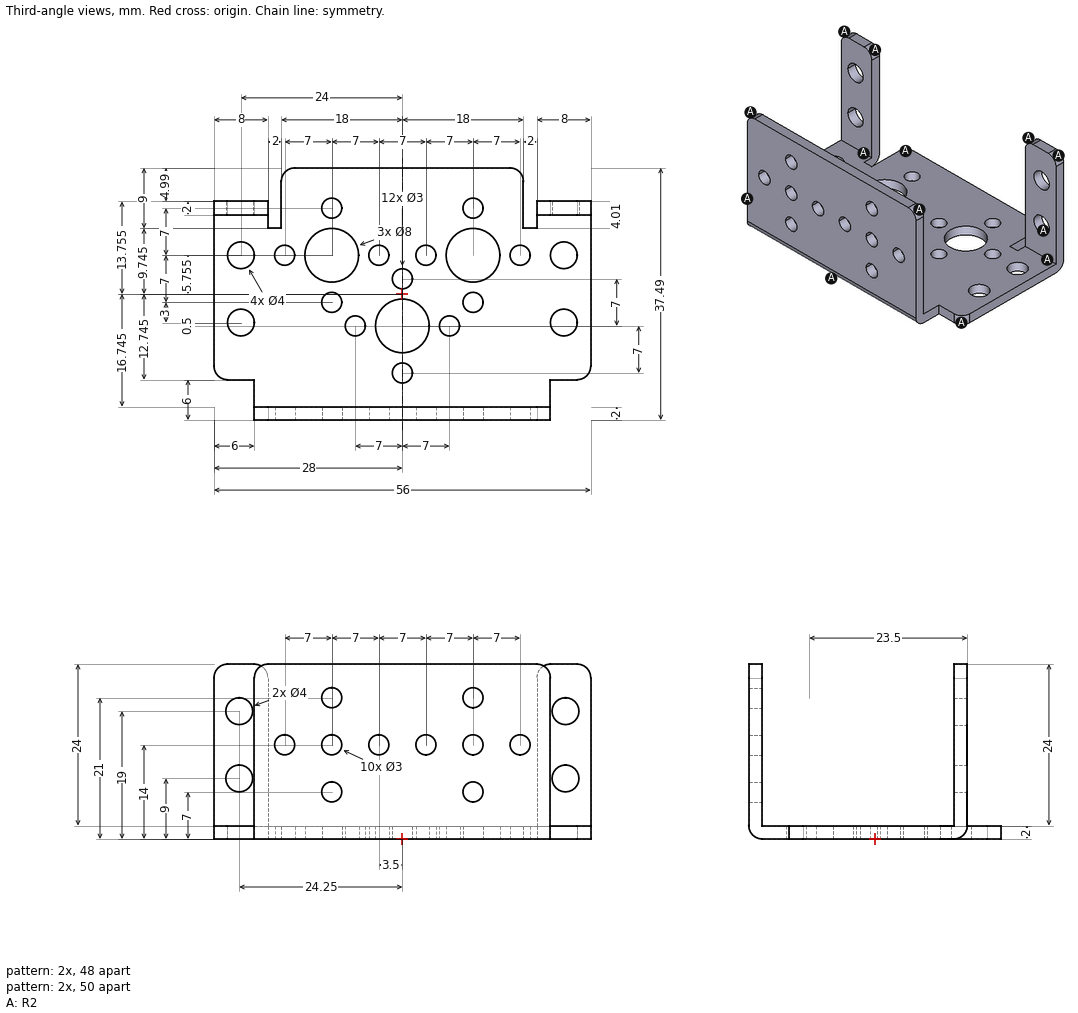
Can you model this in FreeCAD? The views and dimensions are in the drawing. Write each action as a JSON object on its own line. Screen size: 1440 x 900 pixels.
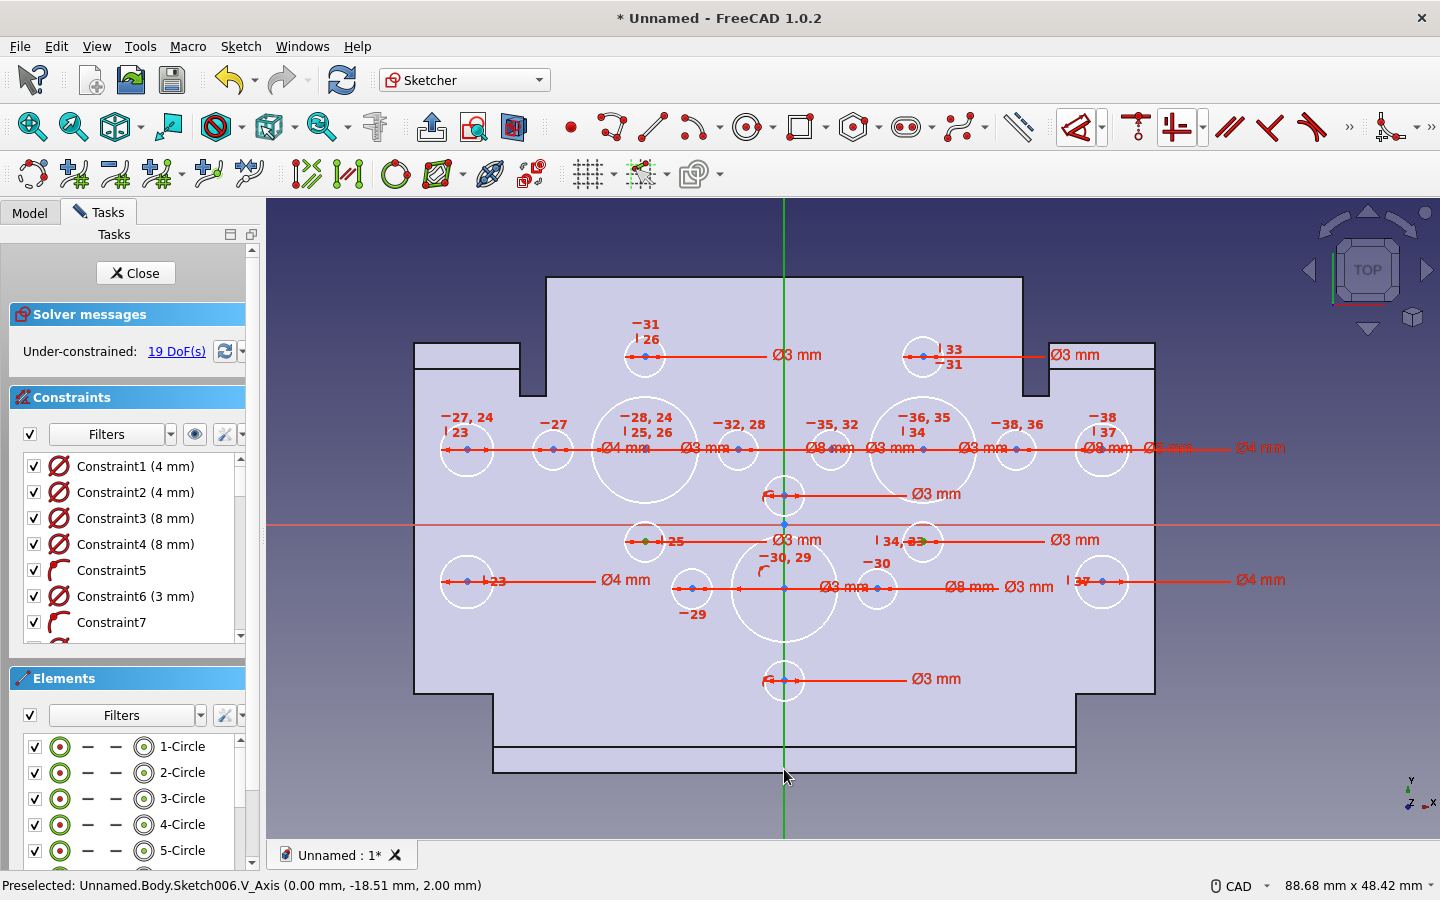
{"action": "key", "text": "s"}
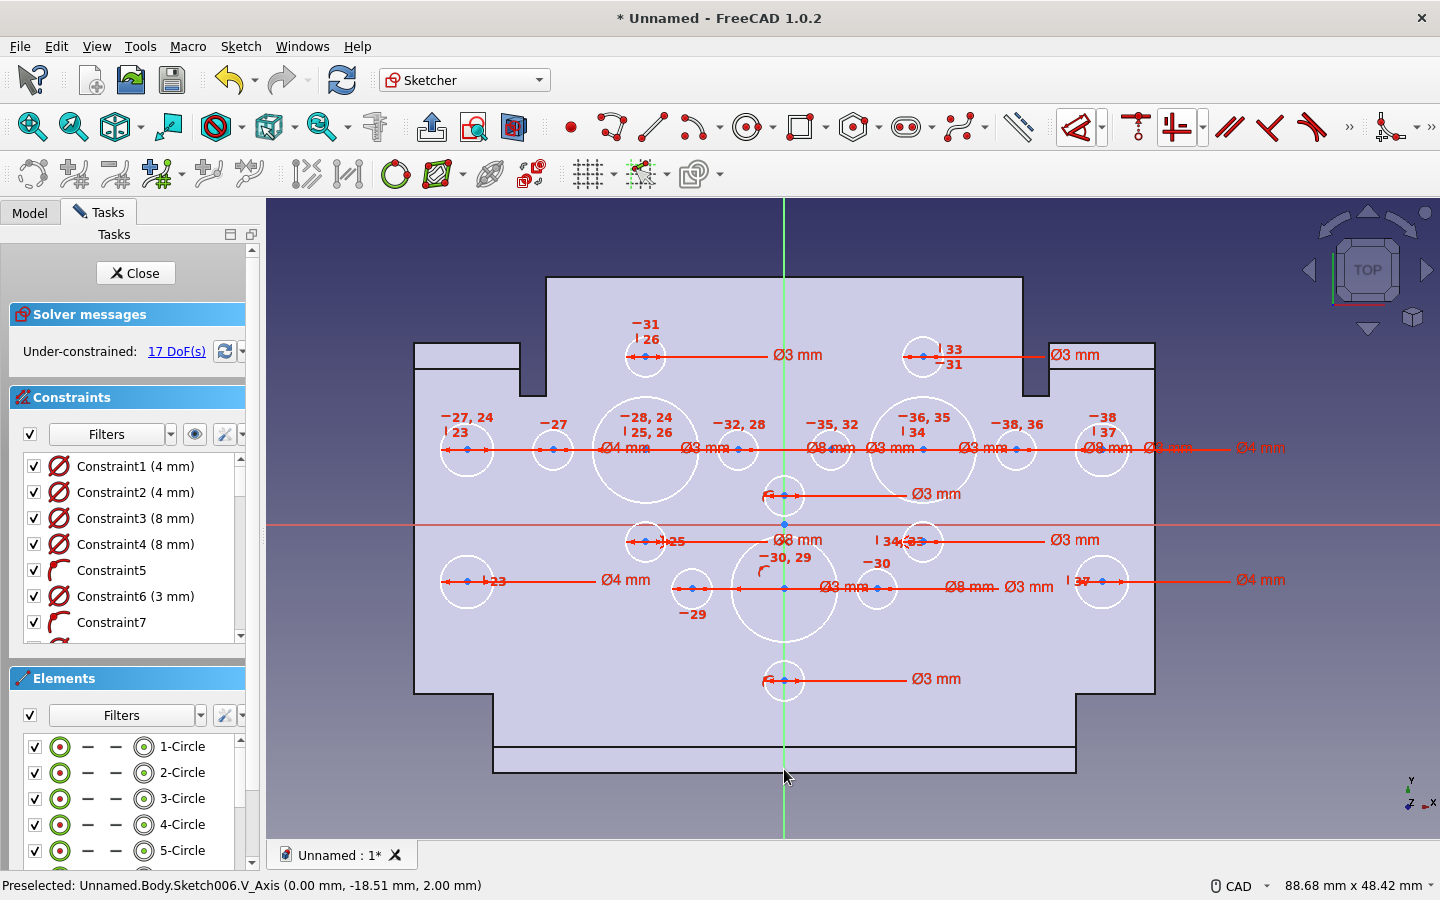
{"action": "left_click", "coordinate": [467, 582]}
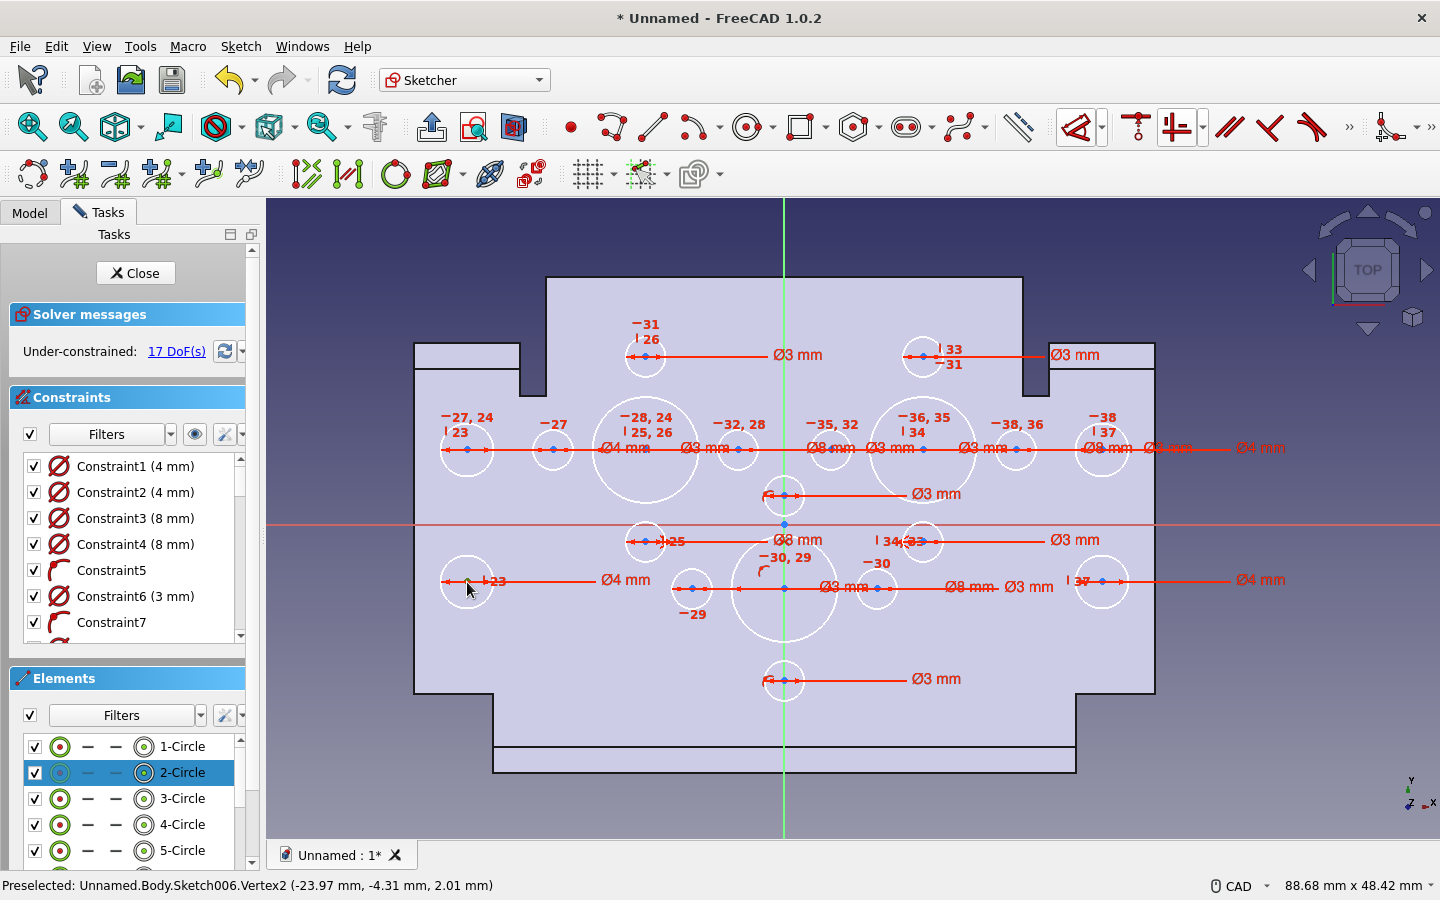
{"action": "left_click", "coordinate": [1102, 582]}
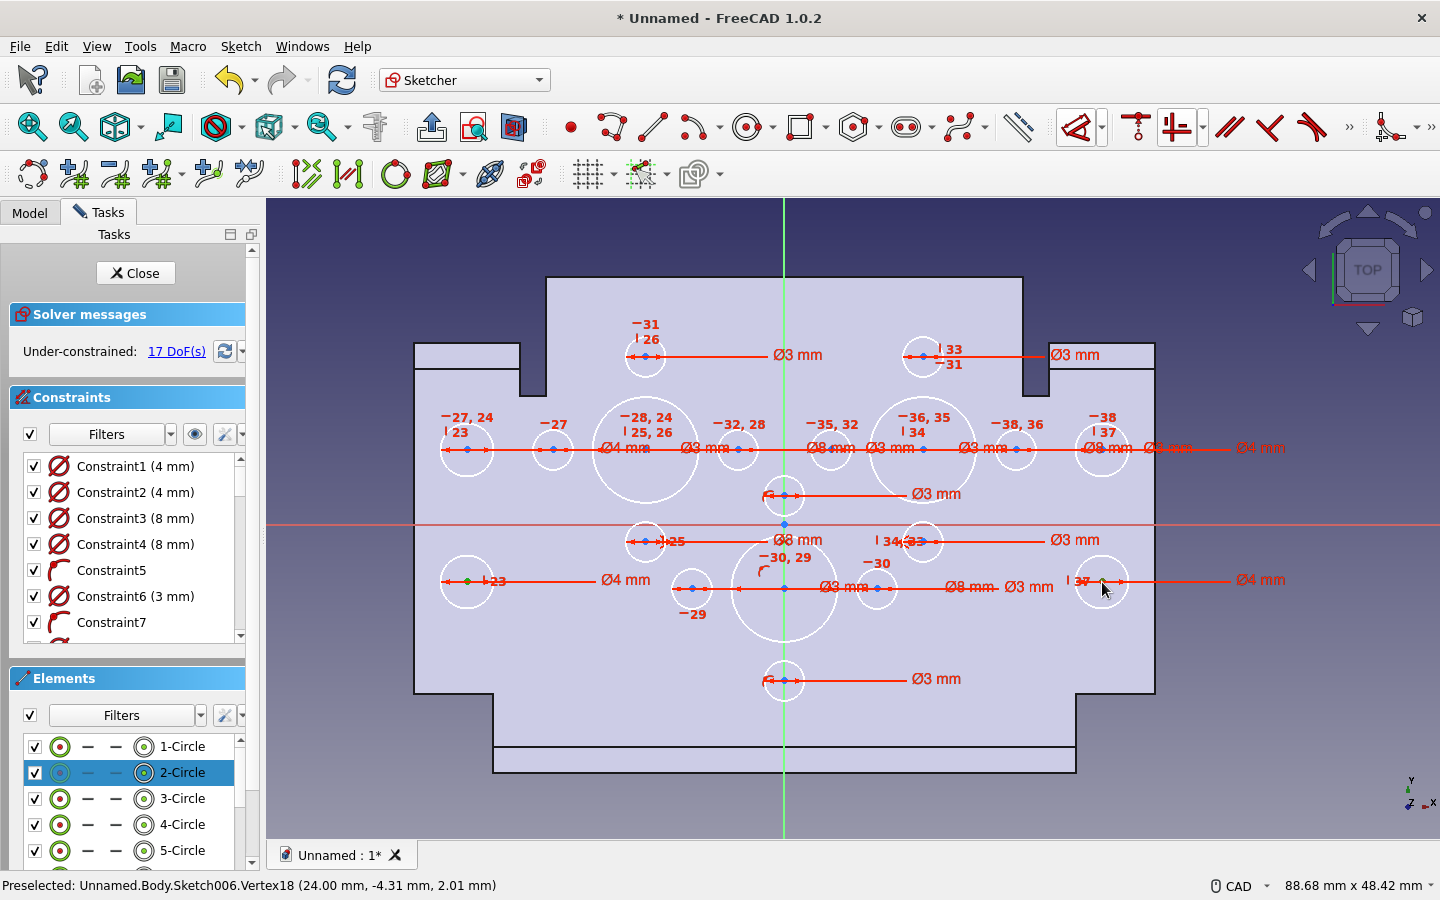
{"action": "left_click", "coordinate": [784, 769]}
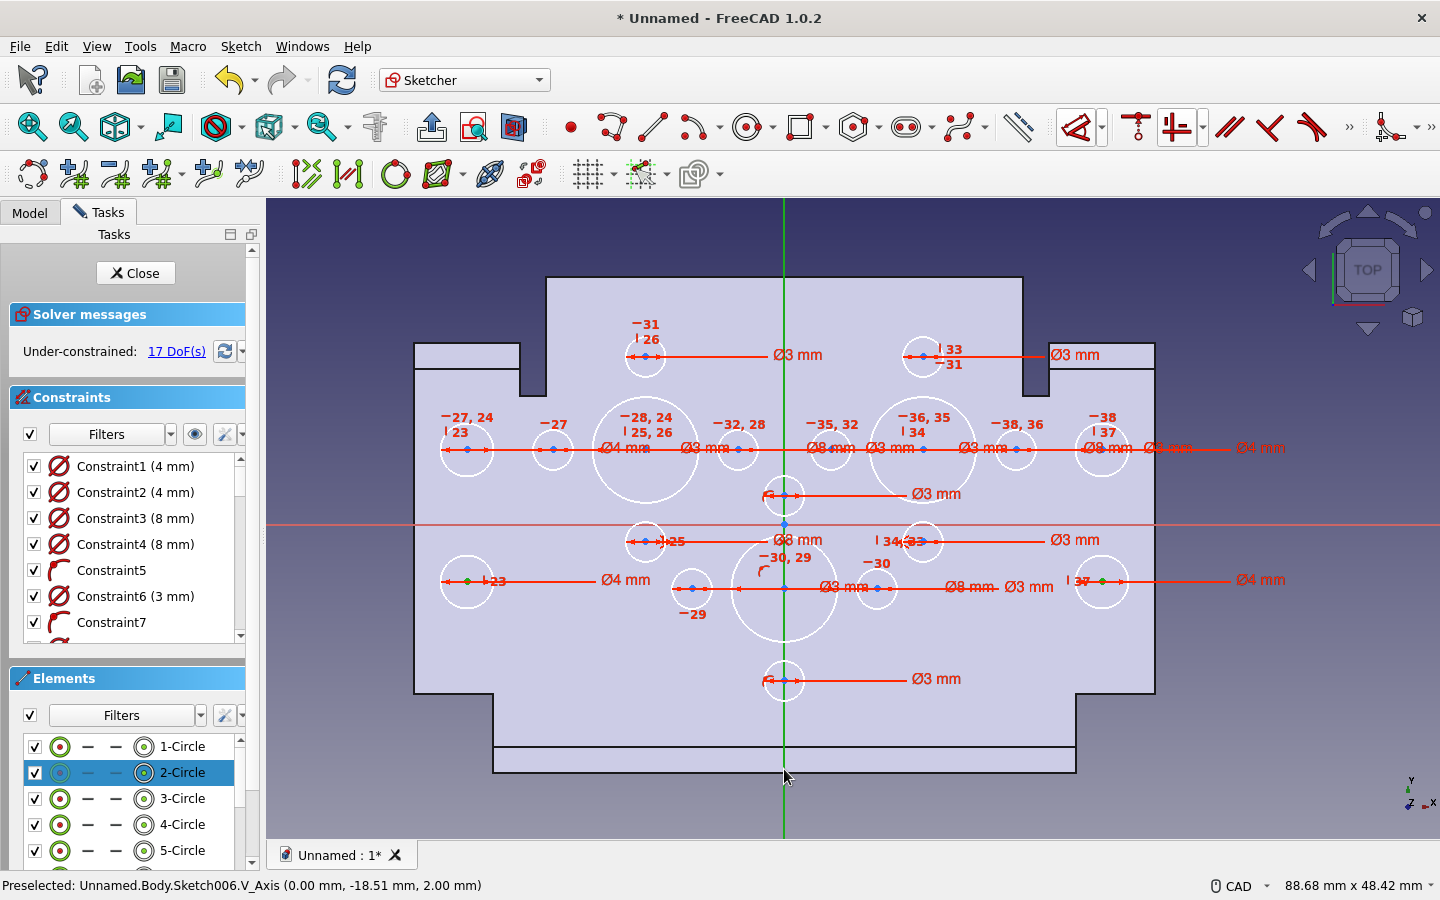
{"action": "key", "text": "s"}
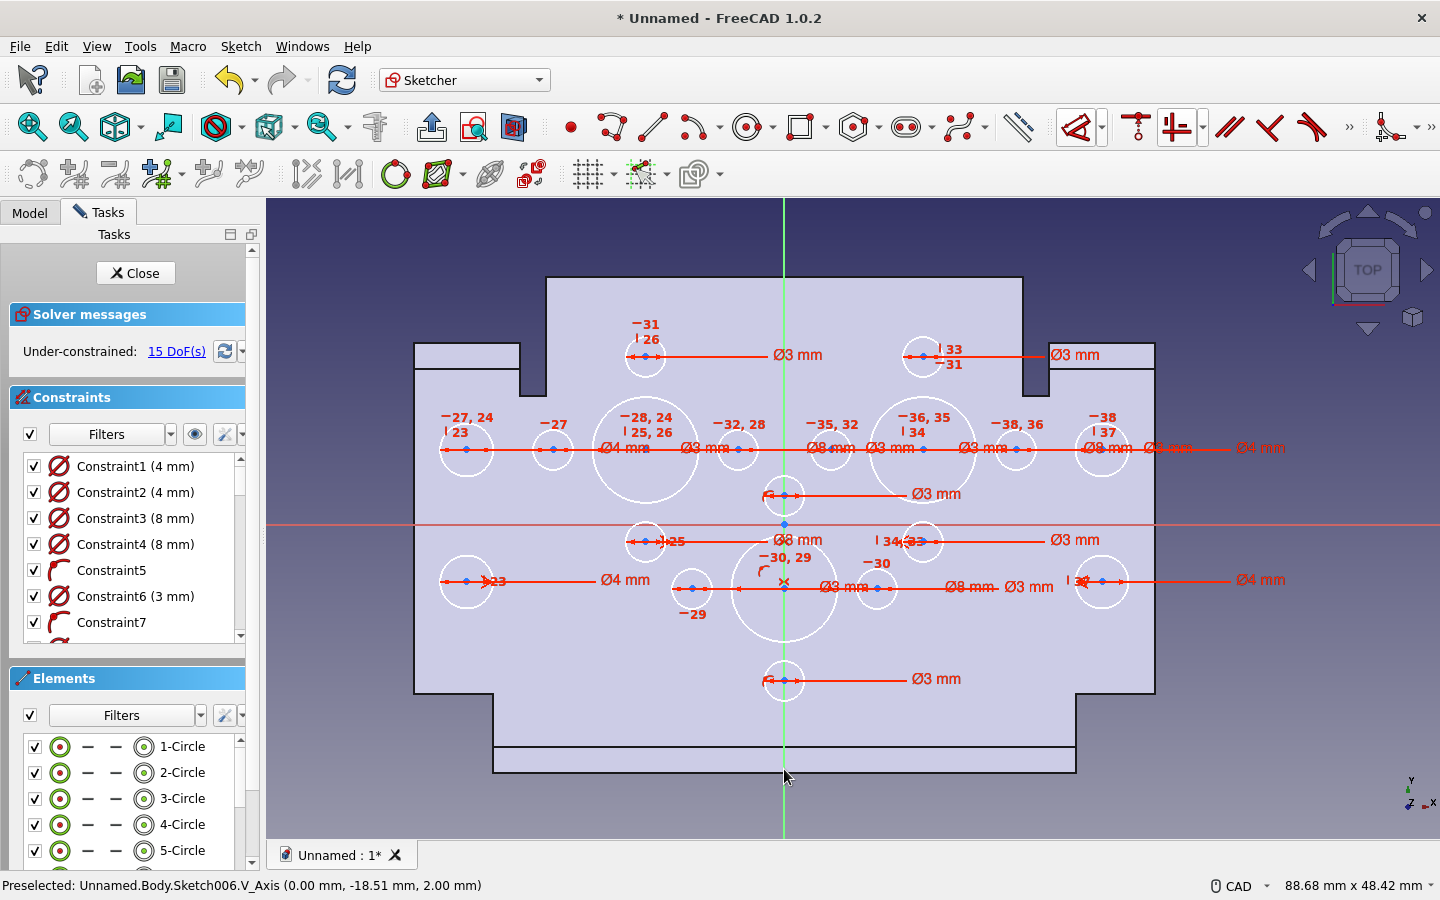
{"action": "left_click", "coordinate": [692, 589]}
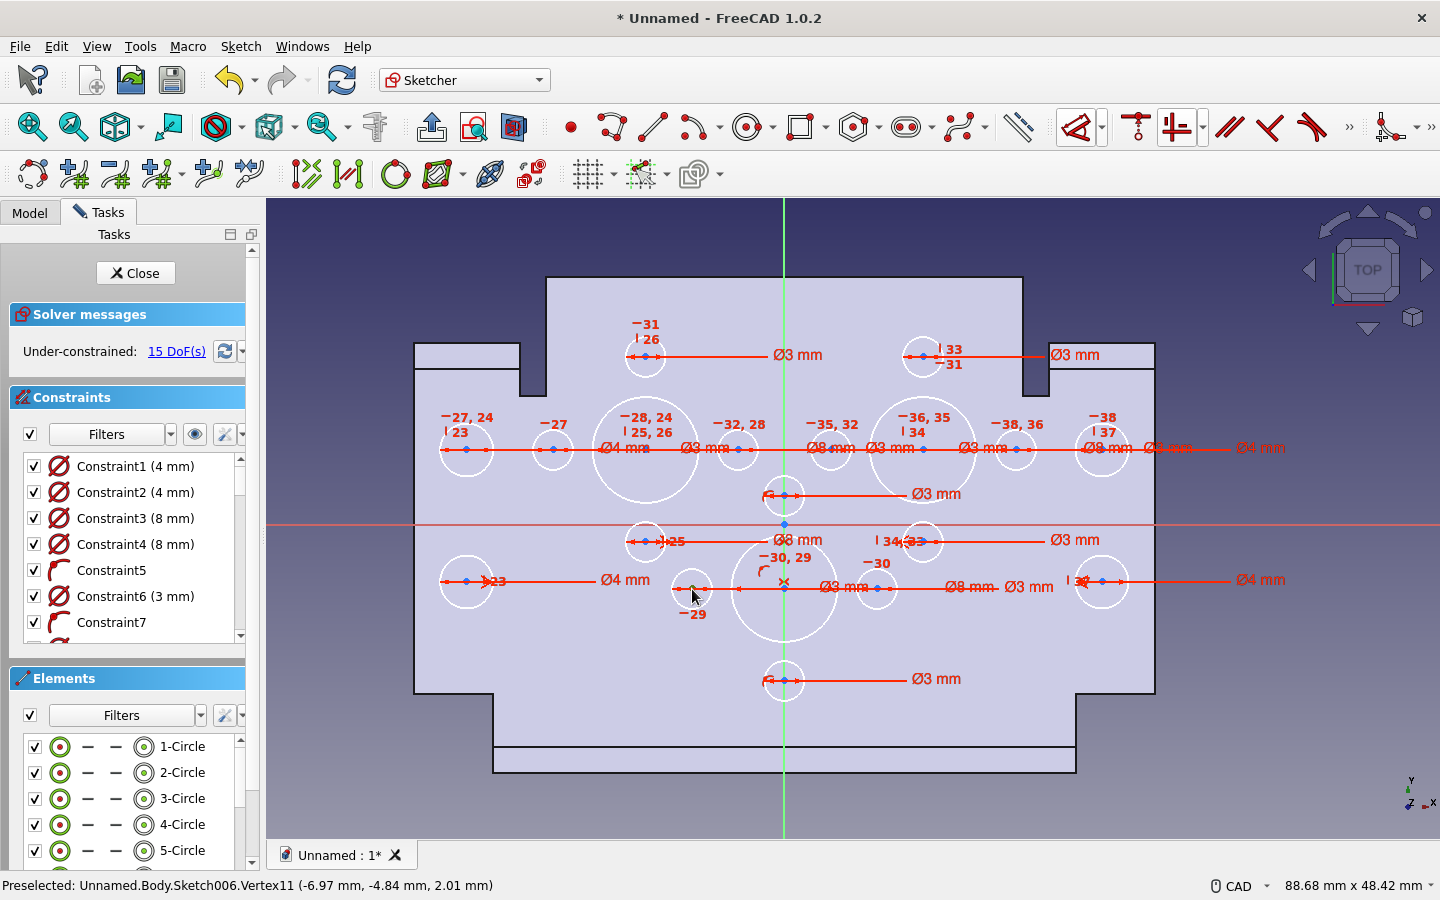
{"action": "key", "text": "l"}